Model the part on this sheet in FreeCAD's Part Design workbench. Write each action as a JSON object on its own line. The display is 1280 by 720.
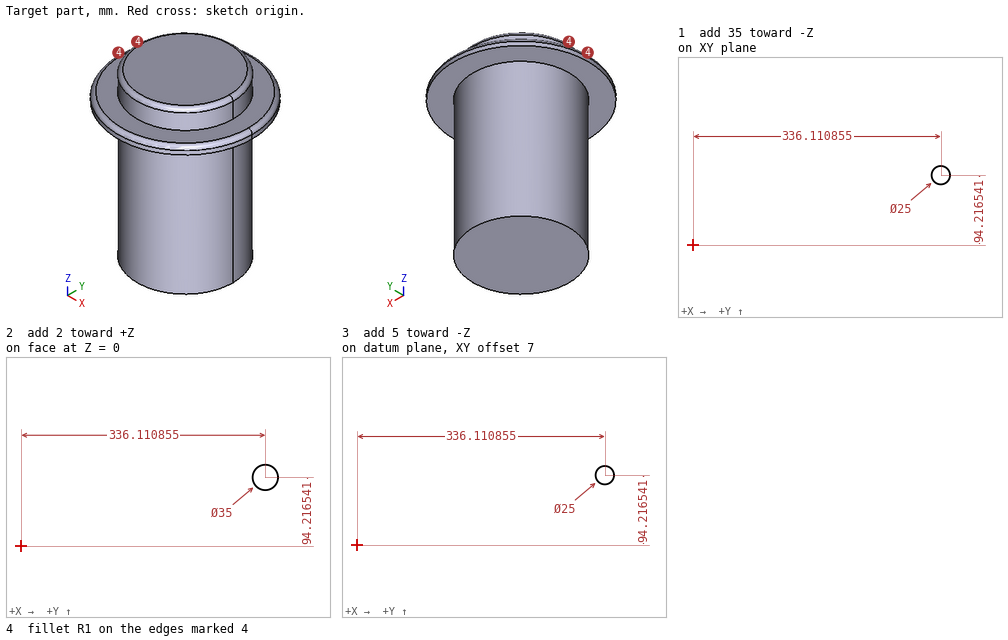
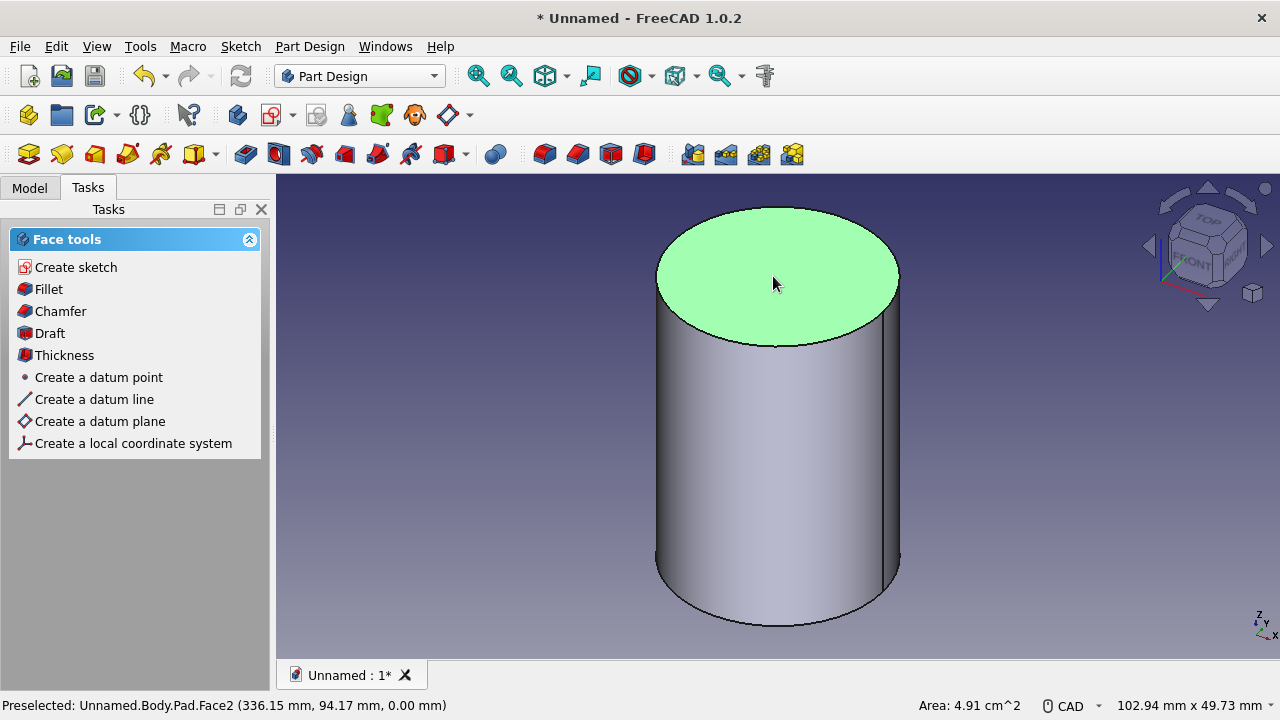
{"action": "left_click", "coordinate": [270, 116]}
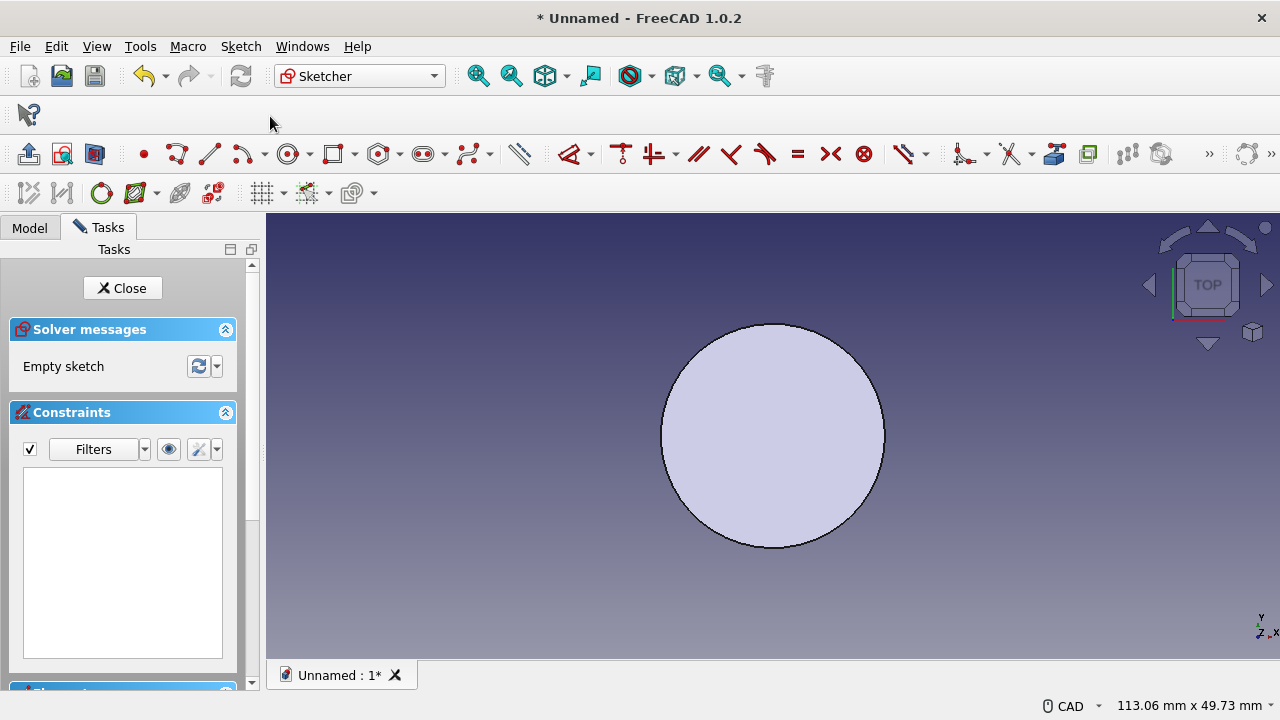
{"action": "left_click", "coordinate": [288, 154]}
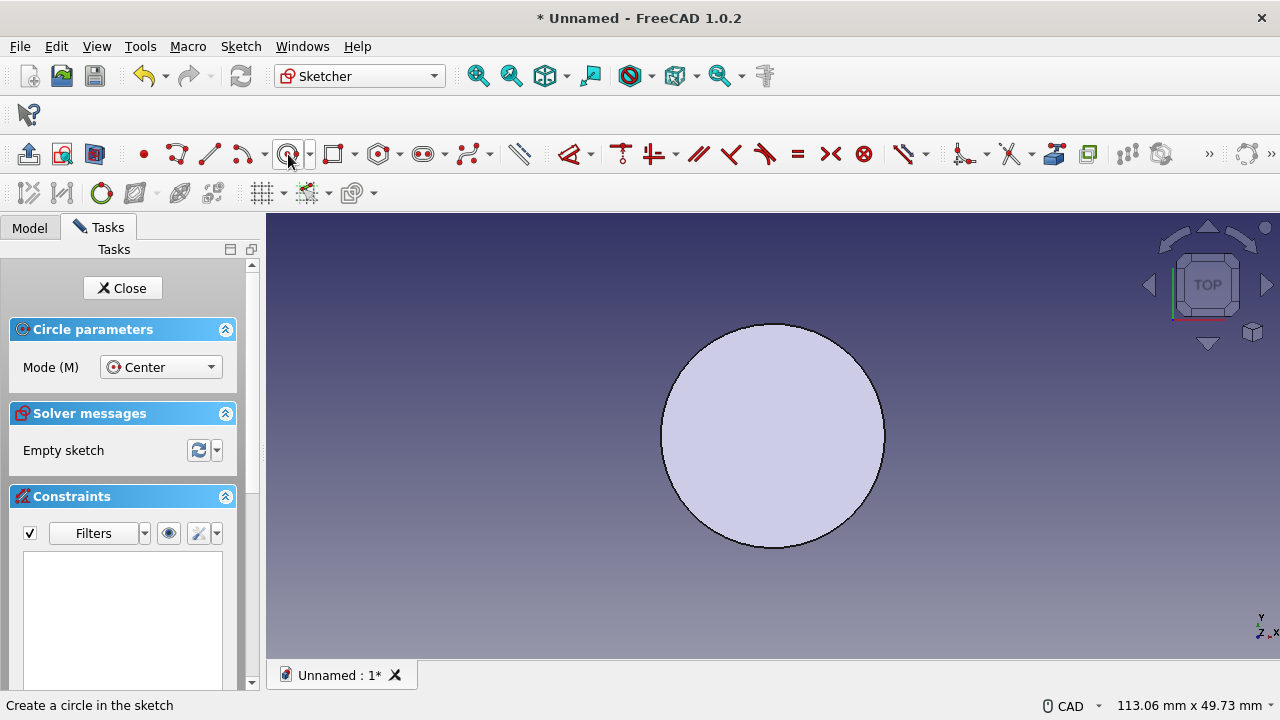
{"action": "left_click", "coordinate": [773, 436]}
{"action": "mouse_move", "coordinate": [884, 325]}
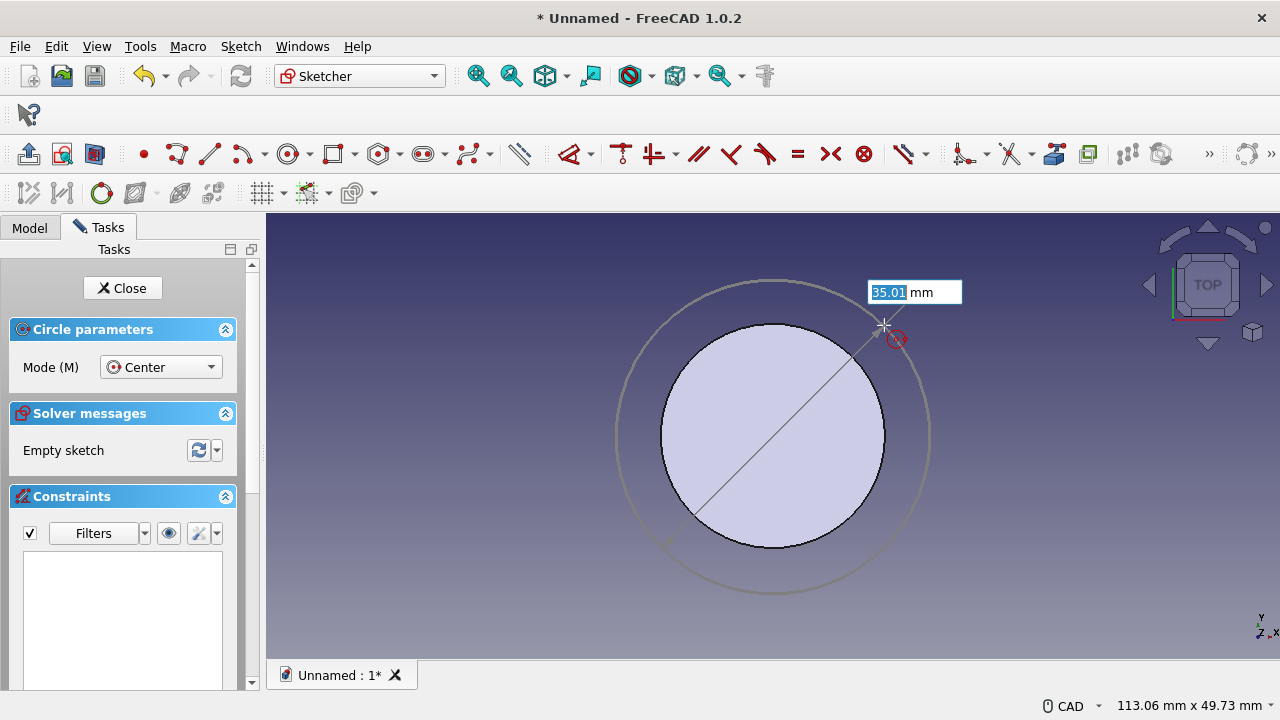
{"action": "type", "text": "35"}
{"action": "key", "text": "Return"}
{"action": "key", "text": "Escape"}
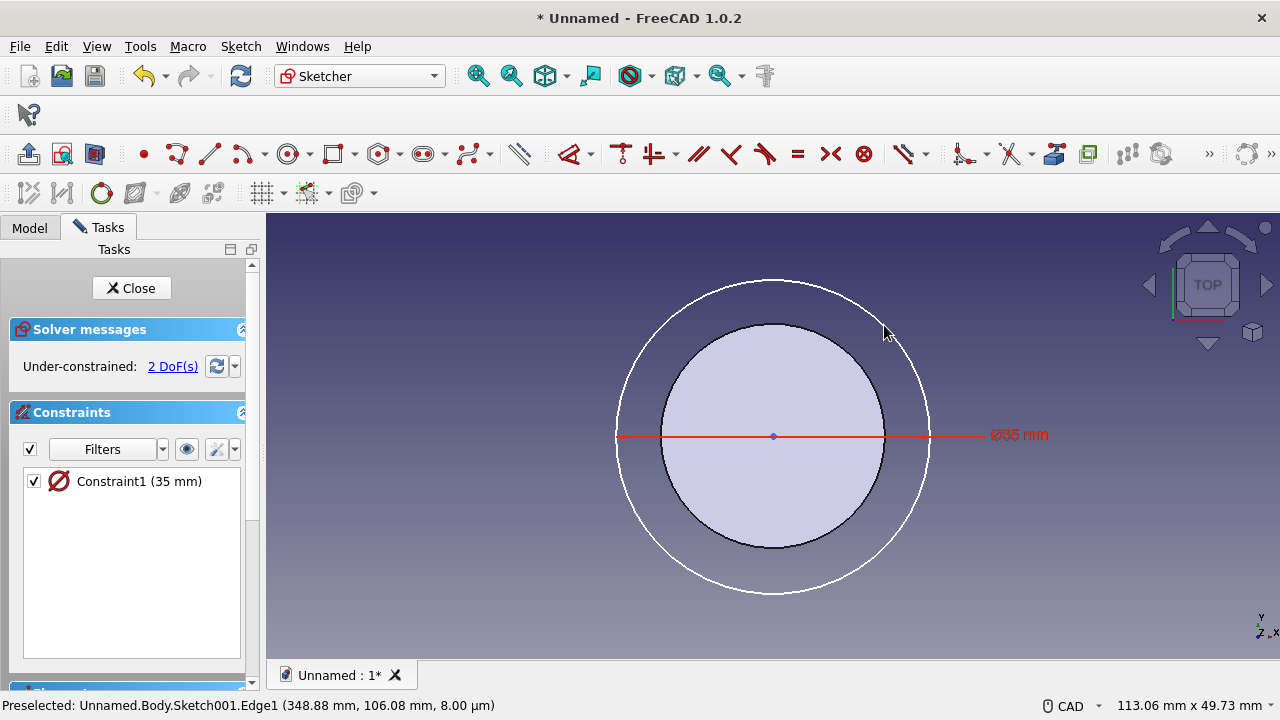
{"action": "left_click", "coordinate": [568, 154]}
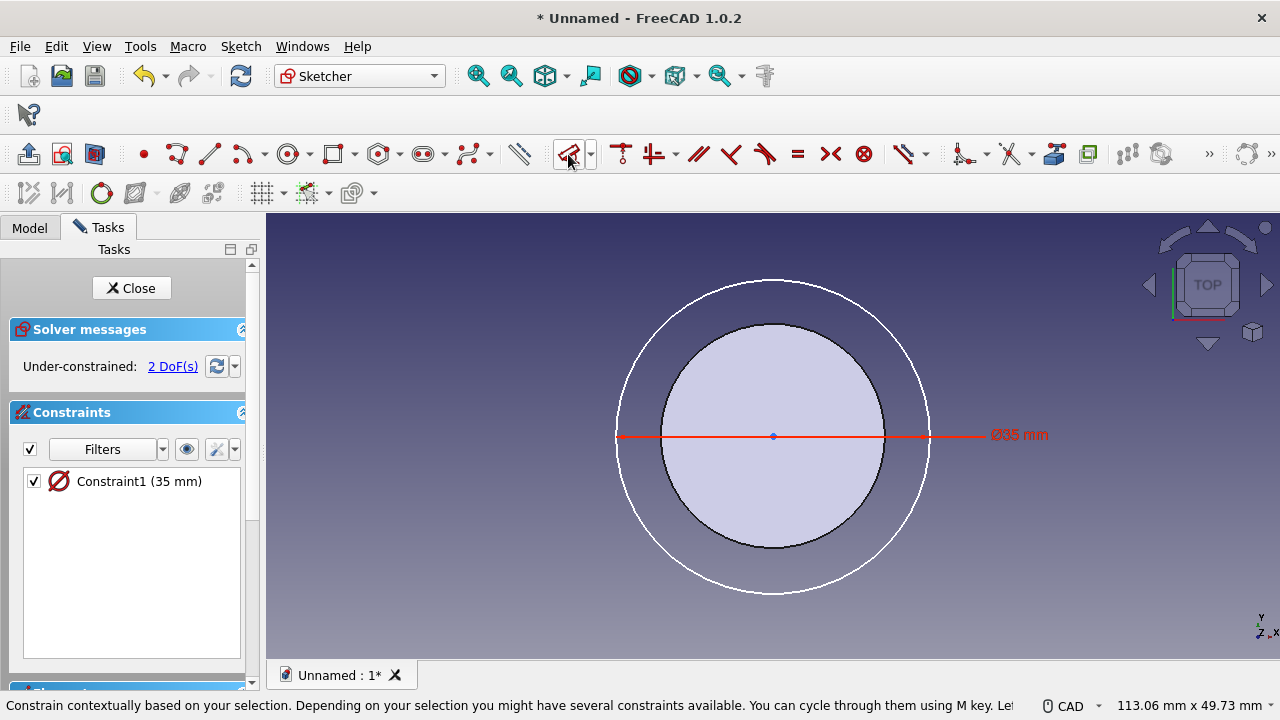
{"action": "left_click", "coordinate": [773, 437]}
{"action": "left_click", "coordinate": [807, 534]}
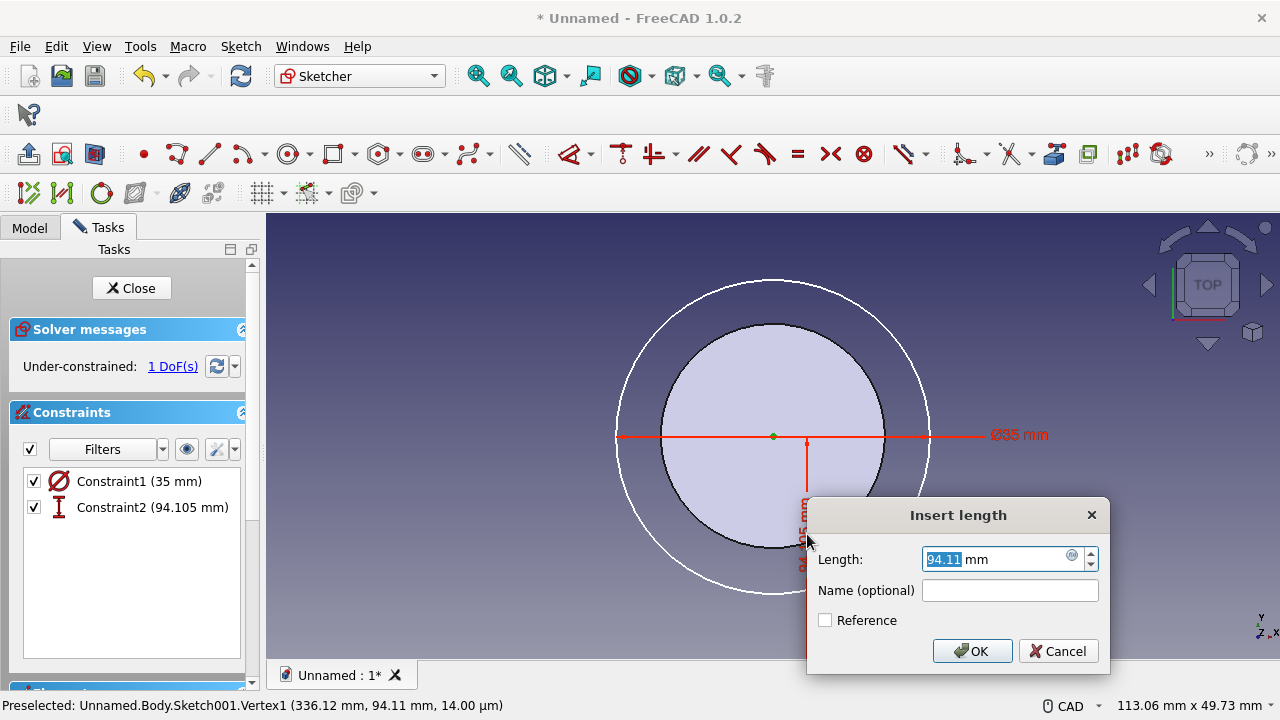
{"action": "type", "text": "94.216541"}
{"action": "key", "text": "Return"}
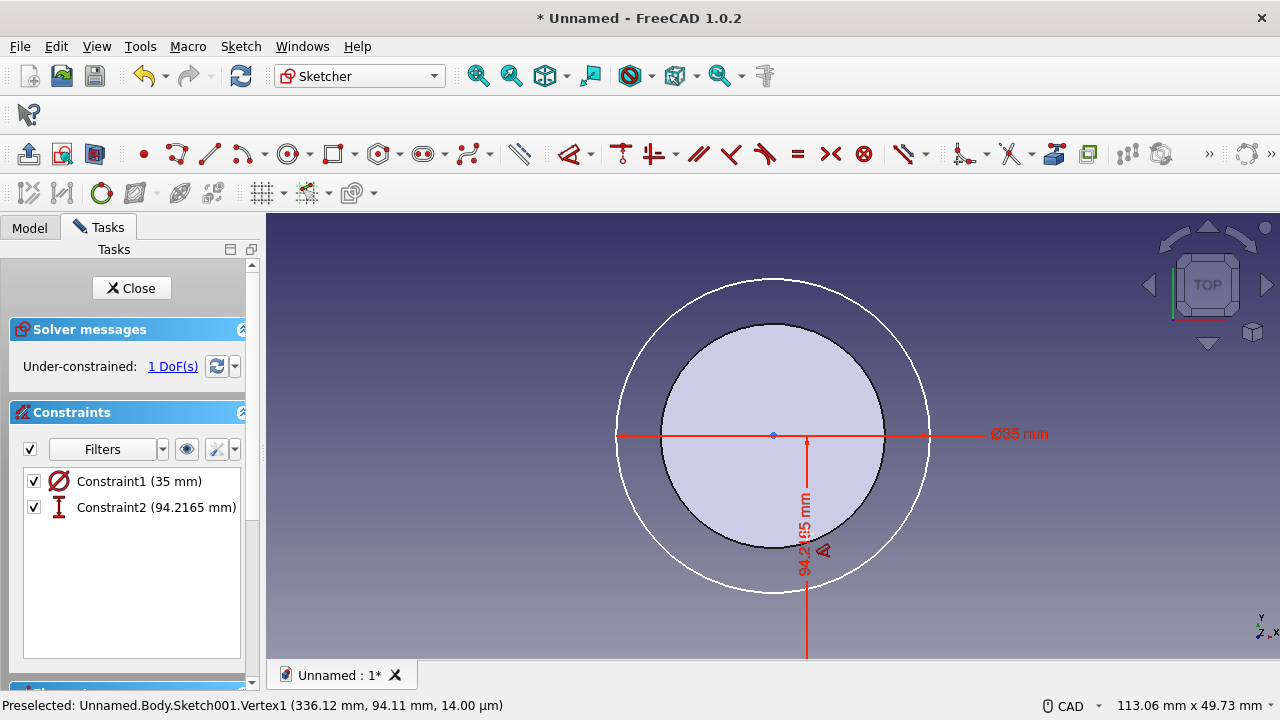
{"action": "left_click", "coordinate": [773, 436]}
{"action": "left_click", "coordinate": [534, 402]}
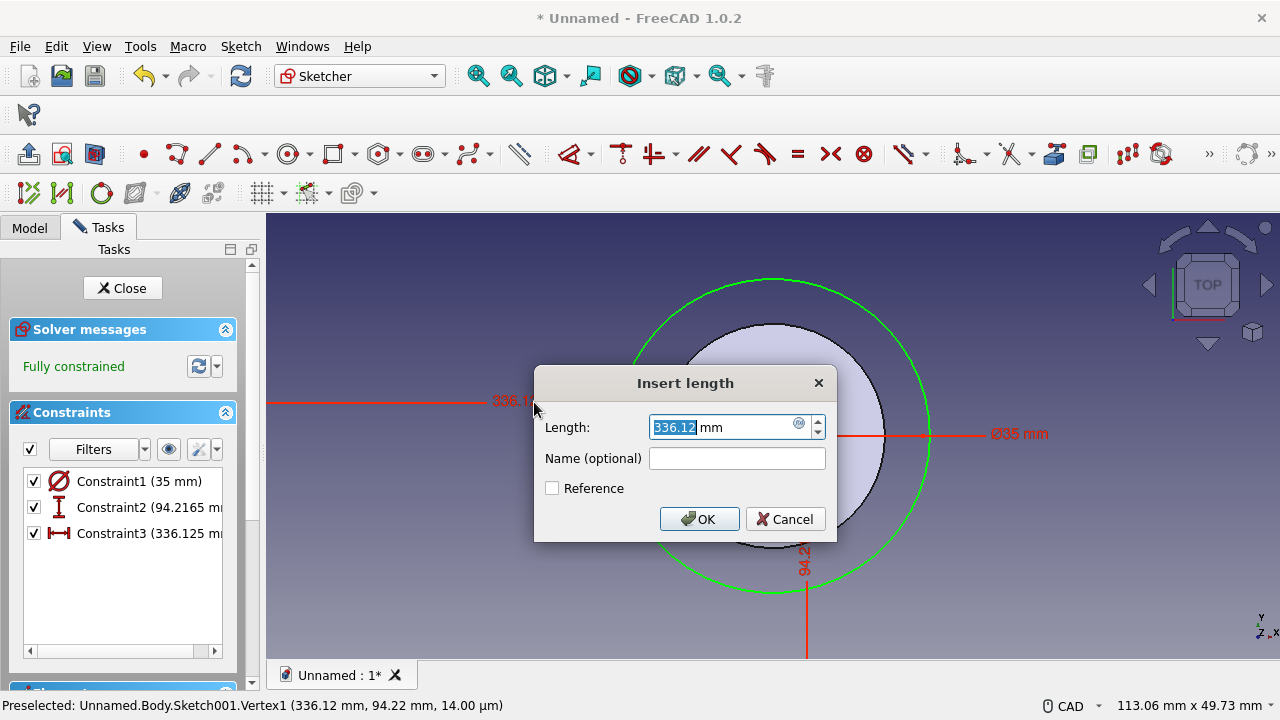
{"action": "type", "text": "336.110855"}
{"action": "key", "text": "Return"}
{"action": "key", "text": "Escape"}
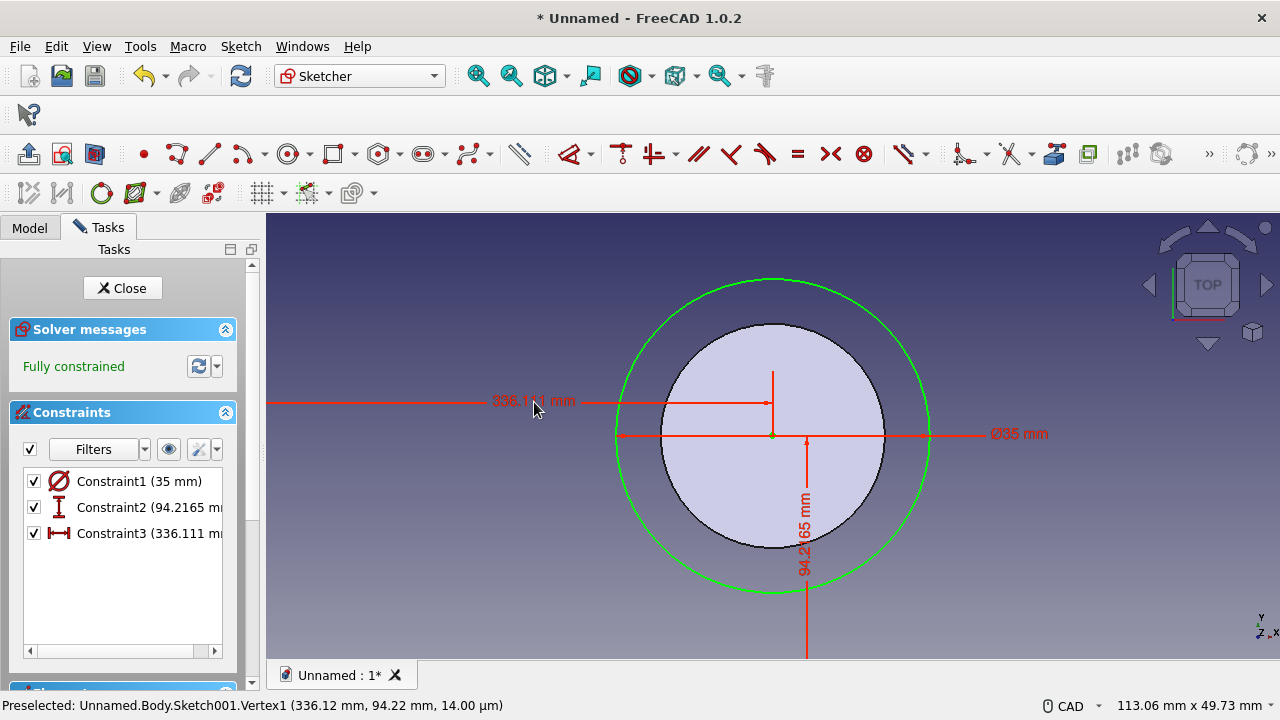
{"action": "left_click", "coordinate": [123, 288]}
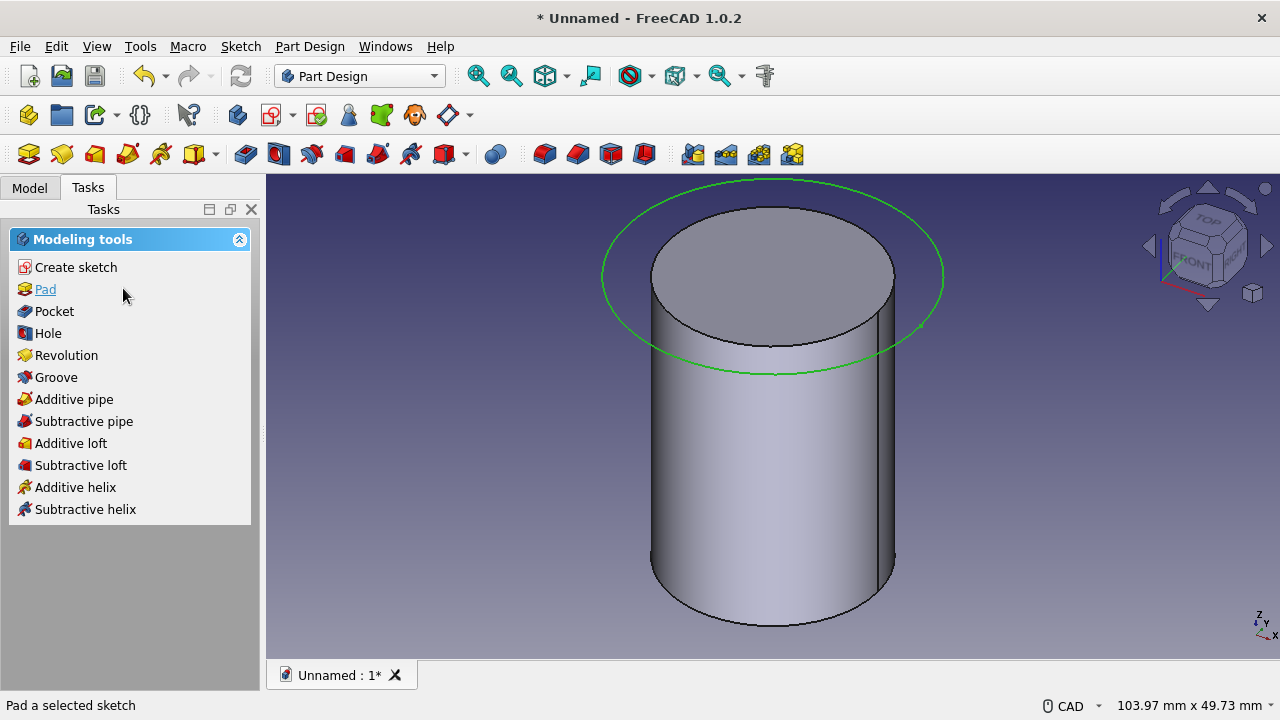
{"action": "left_click", "coordinate": [29, 154]}